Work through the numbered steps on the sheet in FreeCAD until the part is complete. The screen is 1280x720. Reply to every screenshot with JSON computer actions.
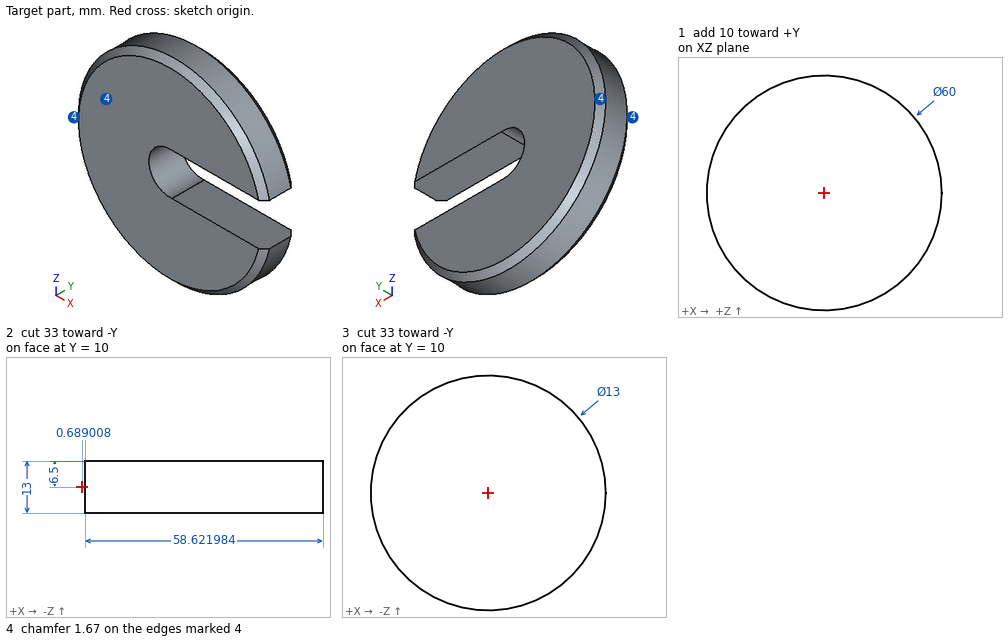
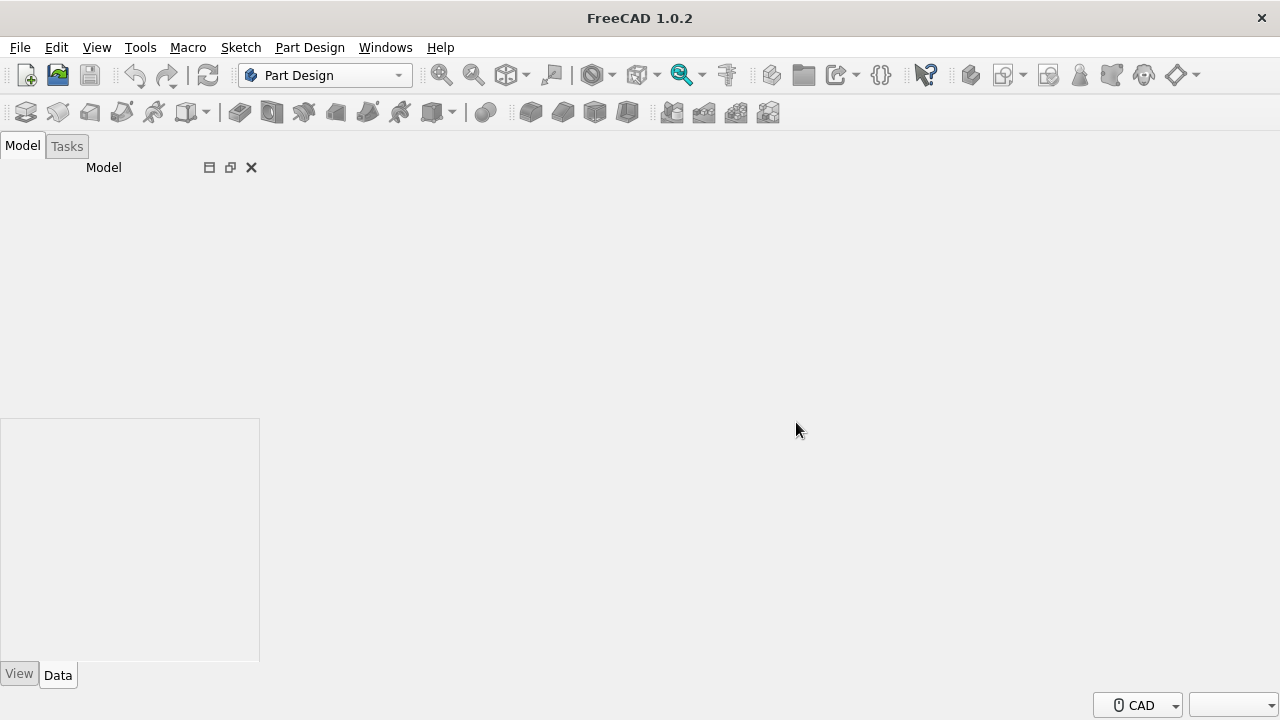
{"action": "left_click", "coordinate": [26, 76]}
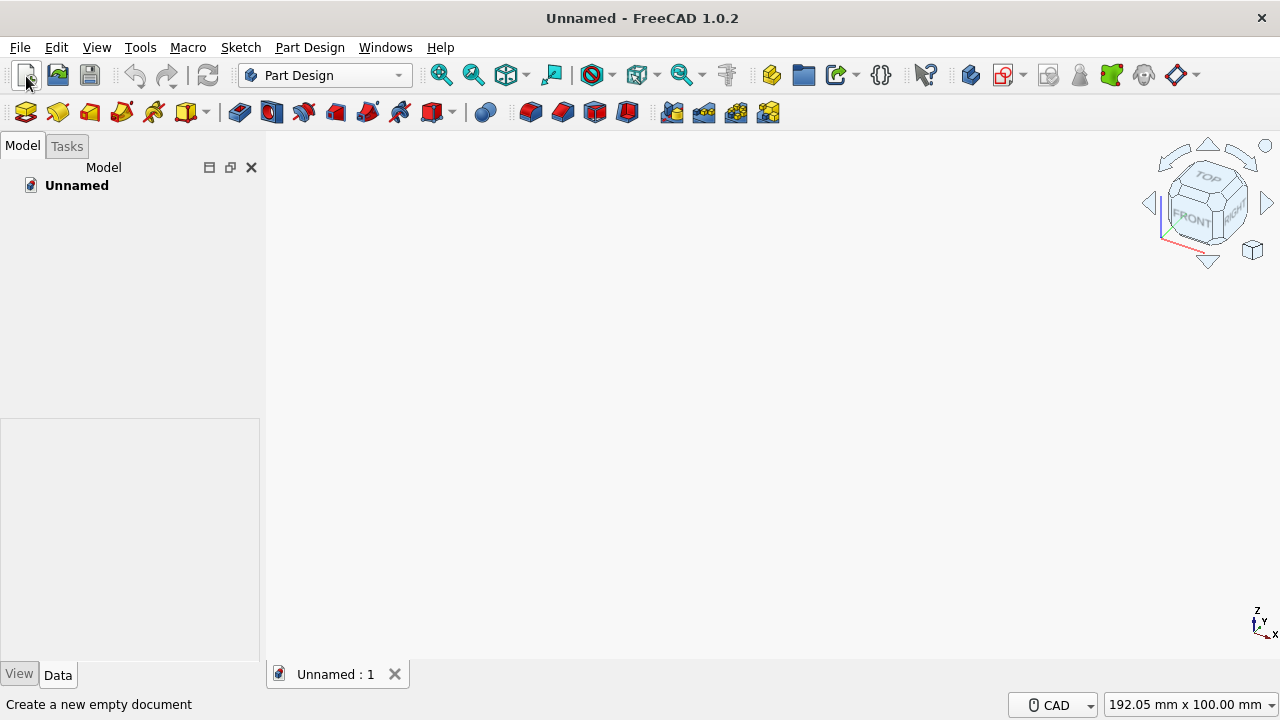
{"action": "left_click", "coordinate": [1004, 76]}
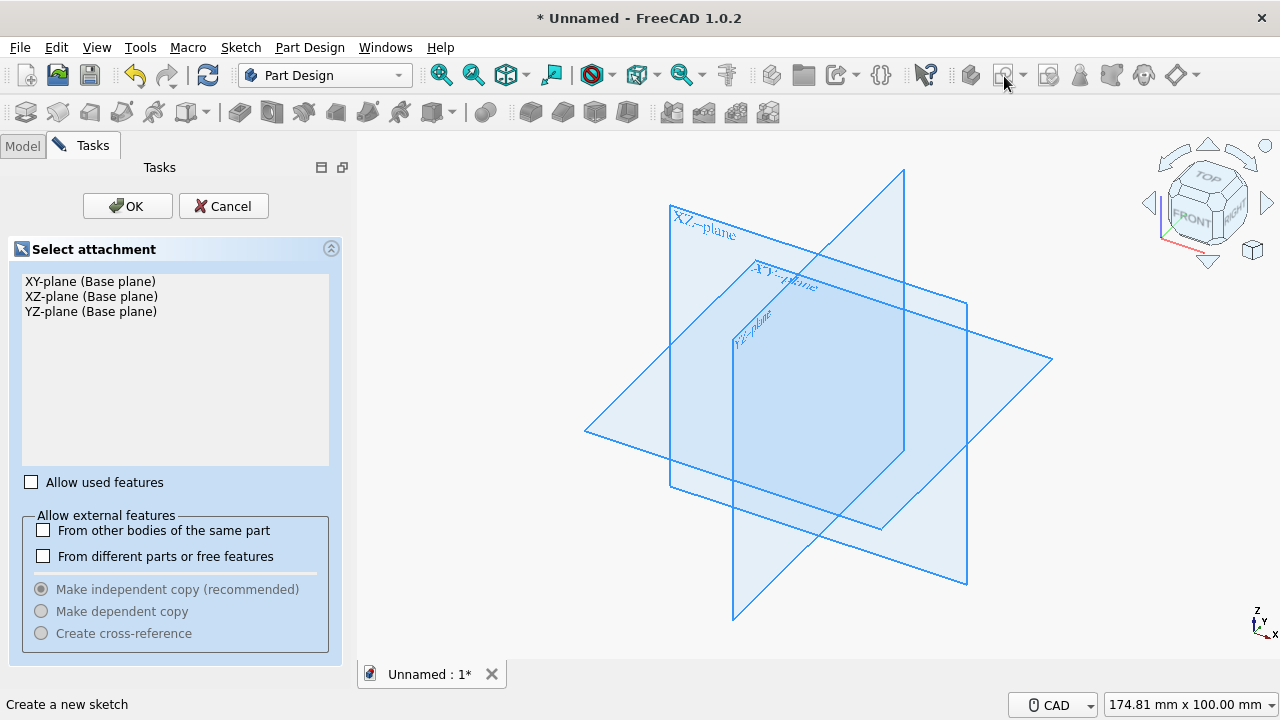
{"action": "left_click", "coordinate": [82, 296]}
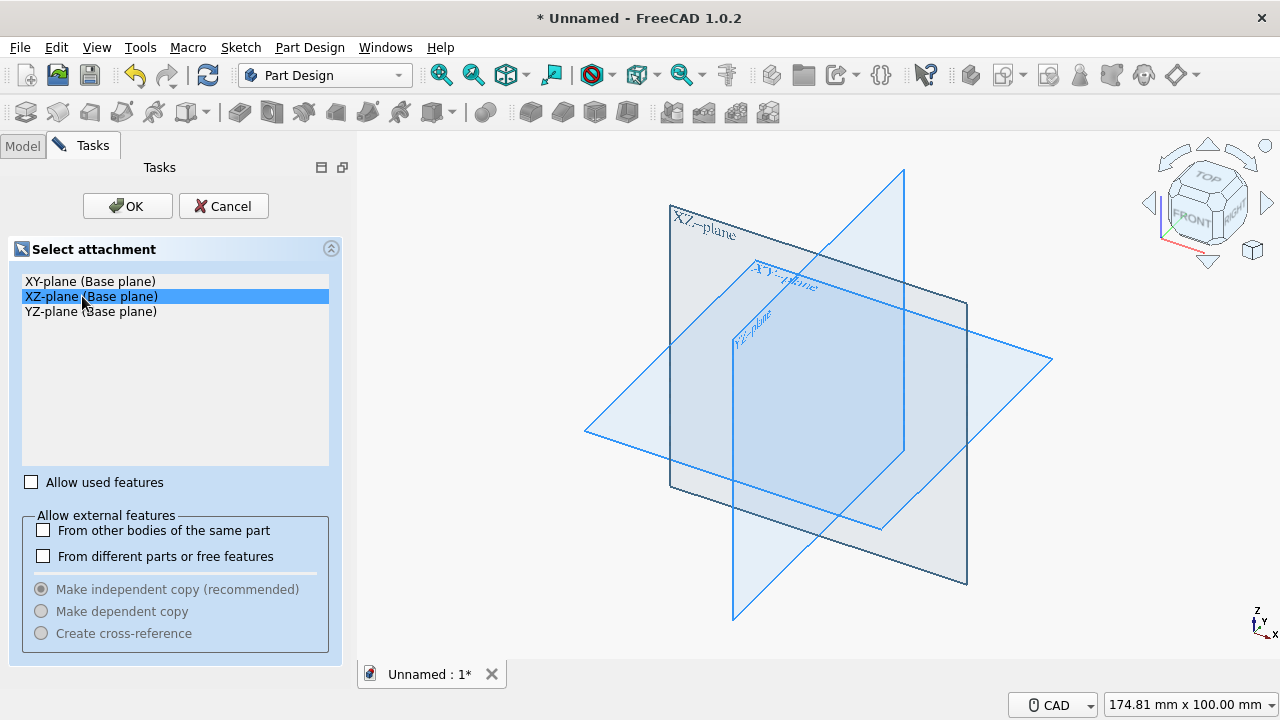
{"action": "left_click", "coordinate": [128, 206]}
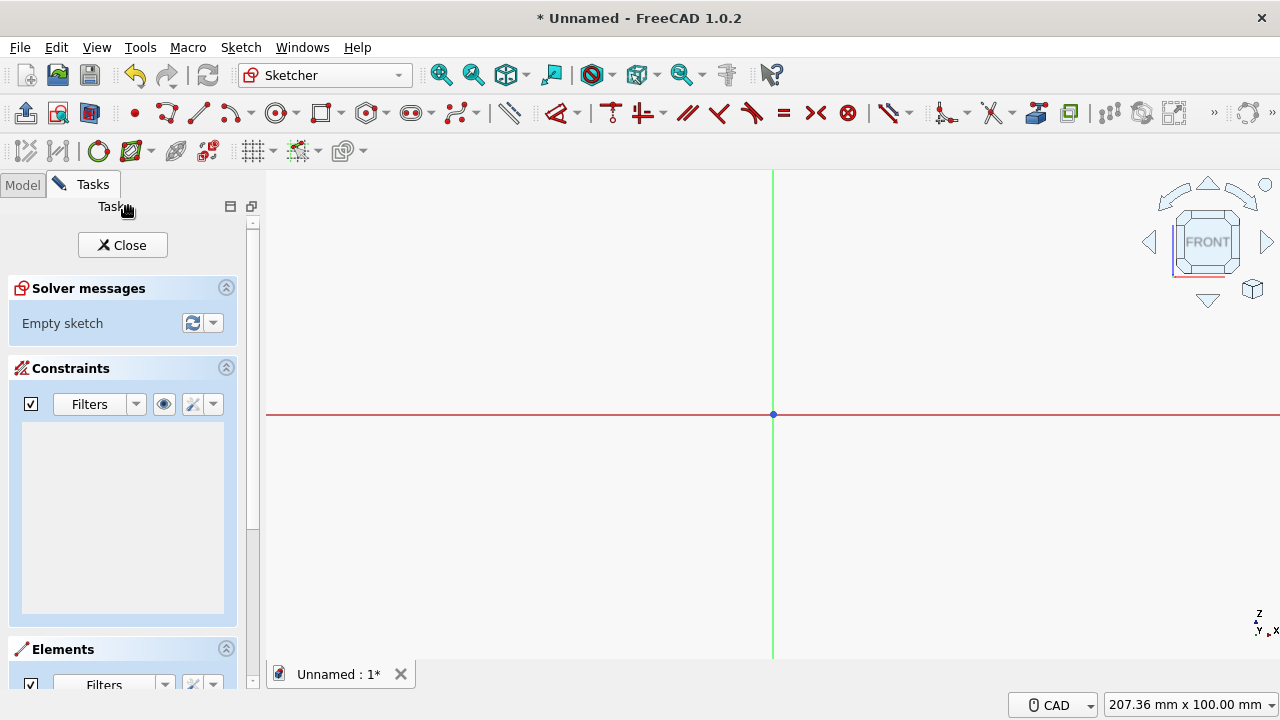
{"action": "key", "text": "g c"}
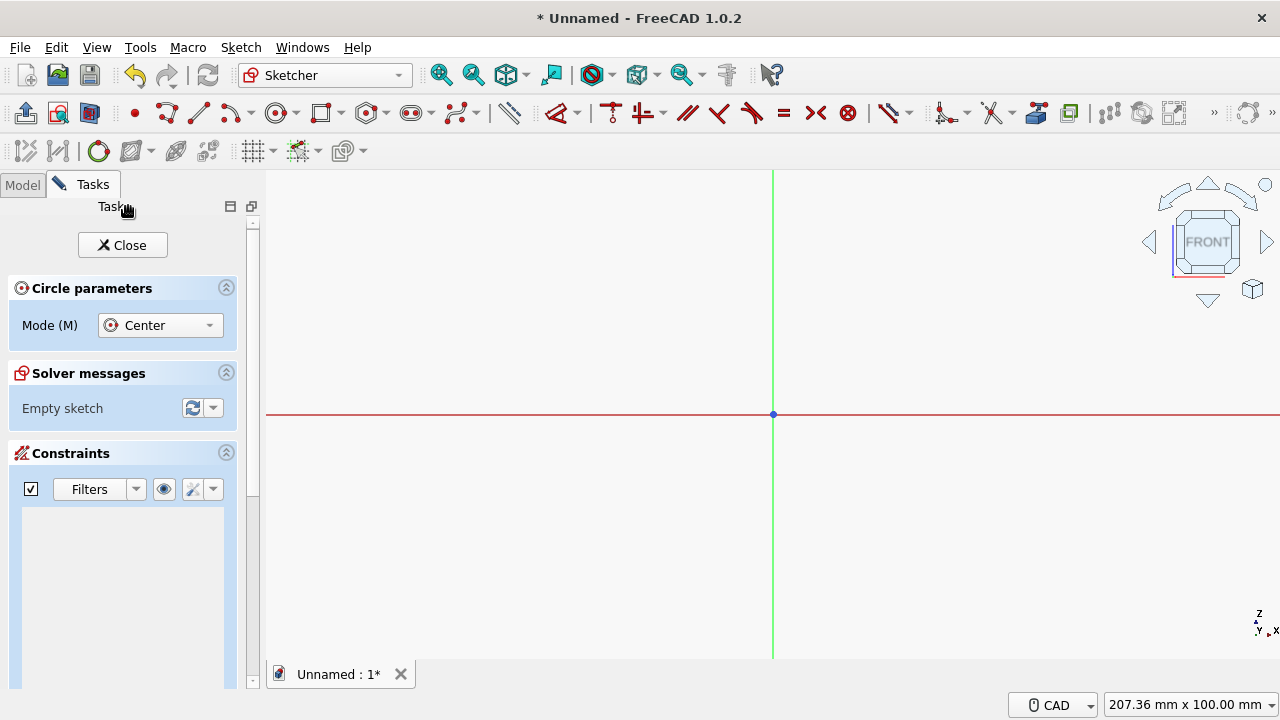
{"action": "left_click", "coordinate": [773, 414]}
{"action": "mouse_move", "coordinate": [877, 311]}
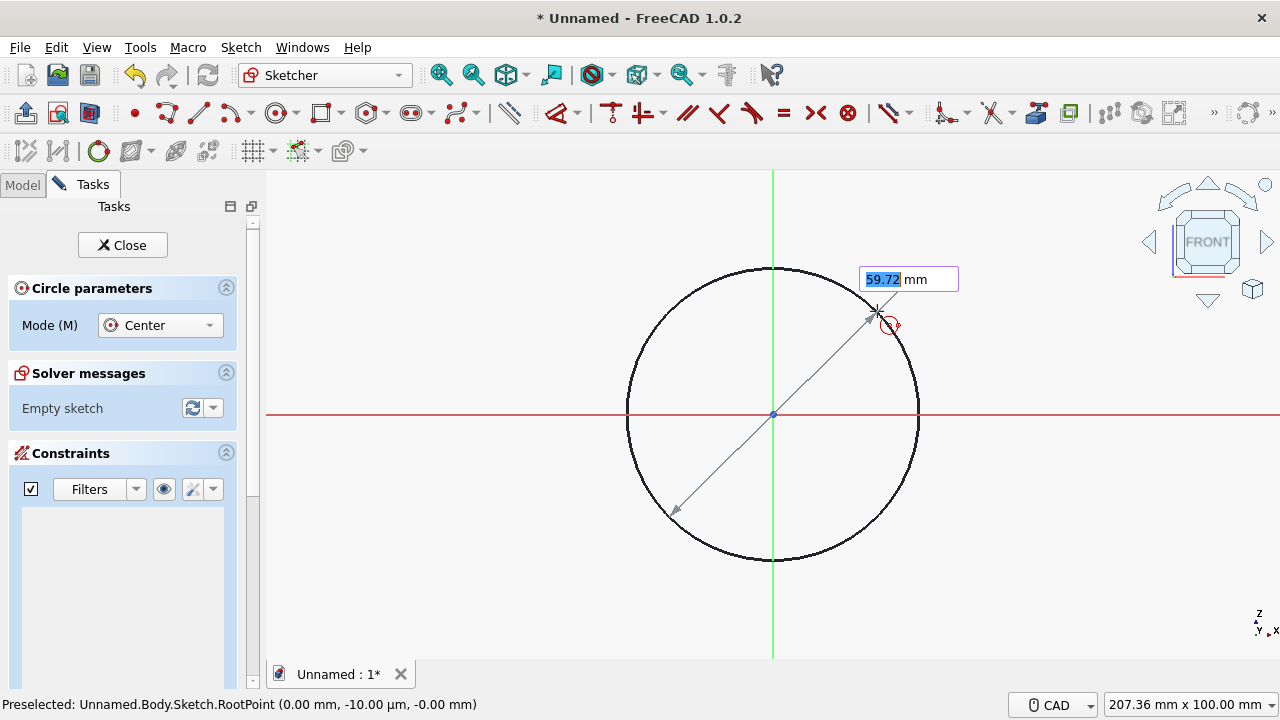
{"action": "type", "text": "60"}
{"action": "key", "text": "Return"}
{"action": "key", "text": "Escape"}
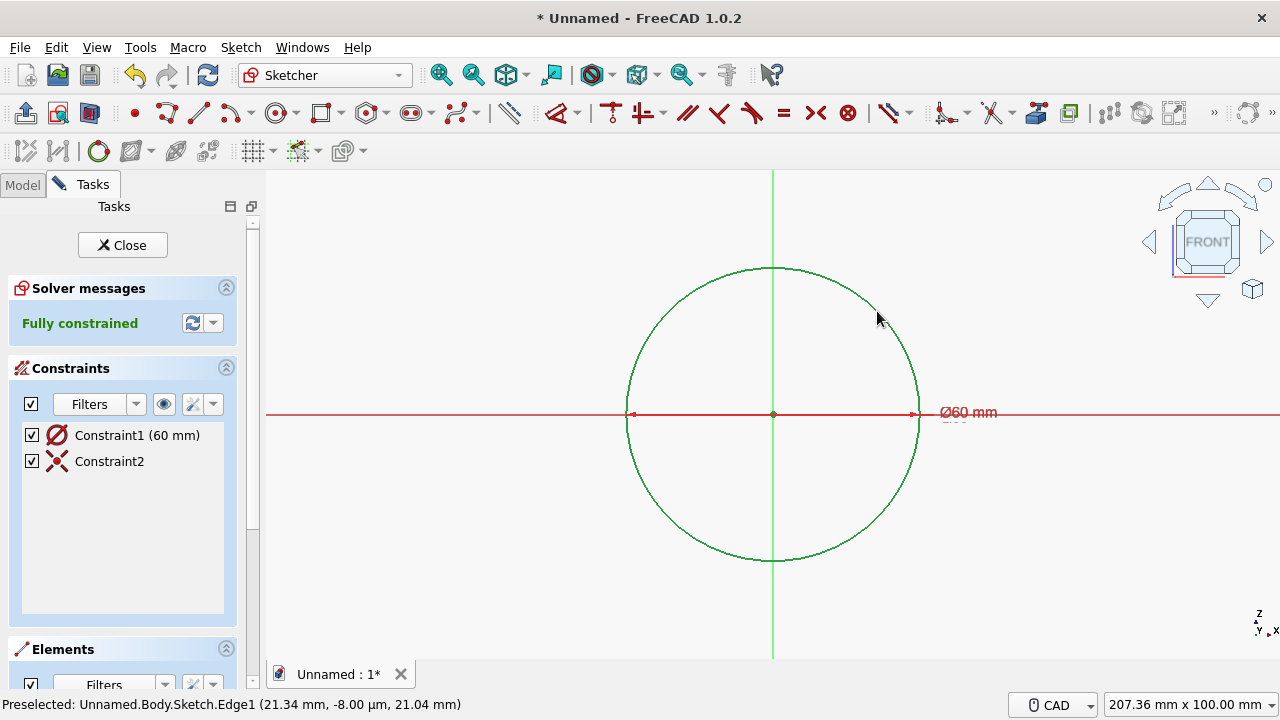
{"action": "left_click", "coordinate": [123, 245]}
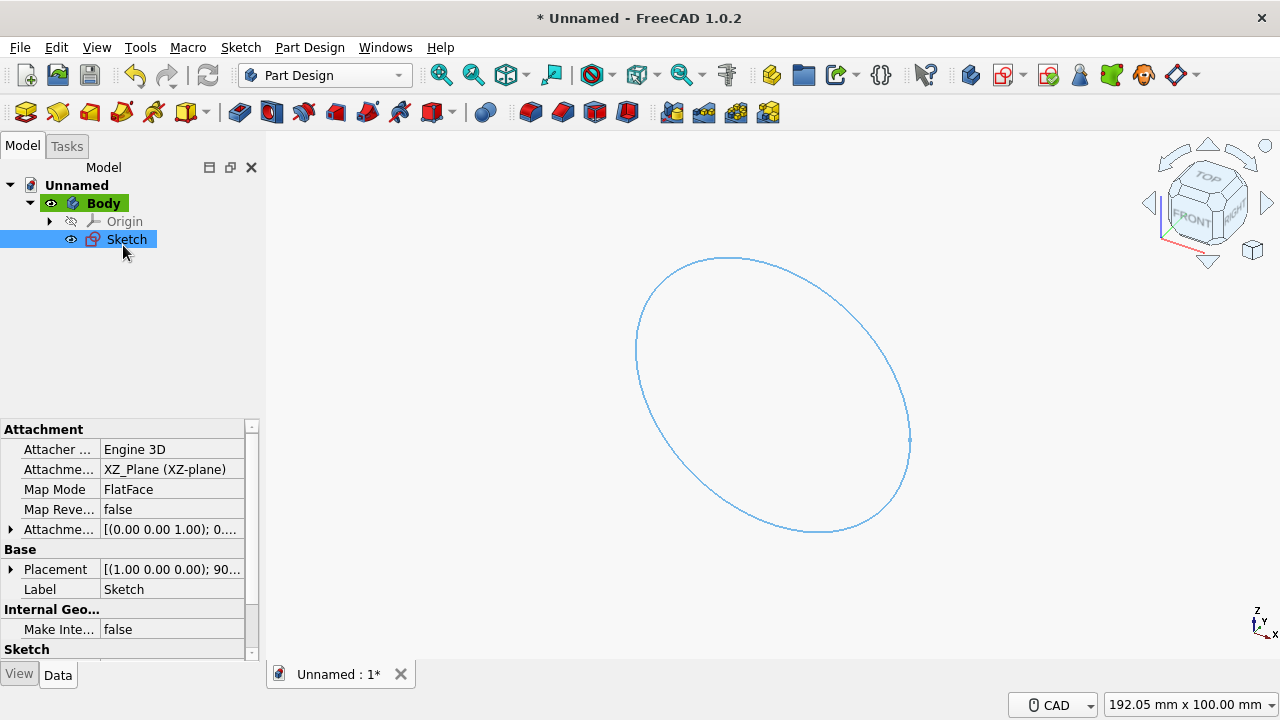
{"action": "left_click", "coordinate": [26, 112]}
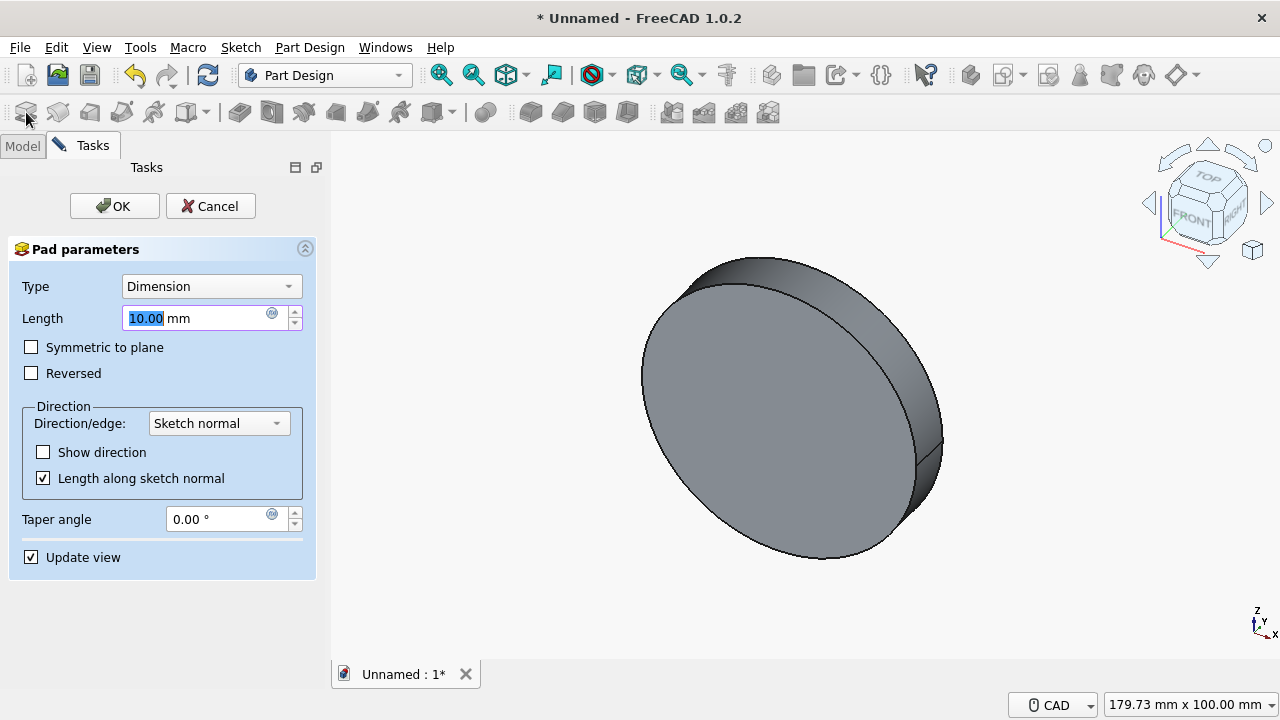
{"action": "type", "text": "10"}
{"action": "key", "text": "Tab"}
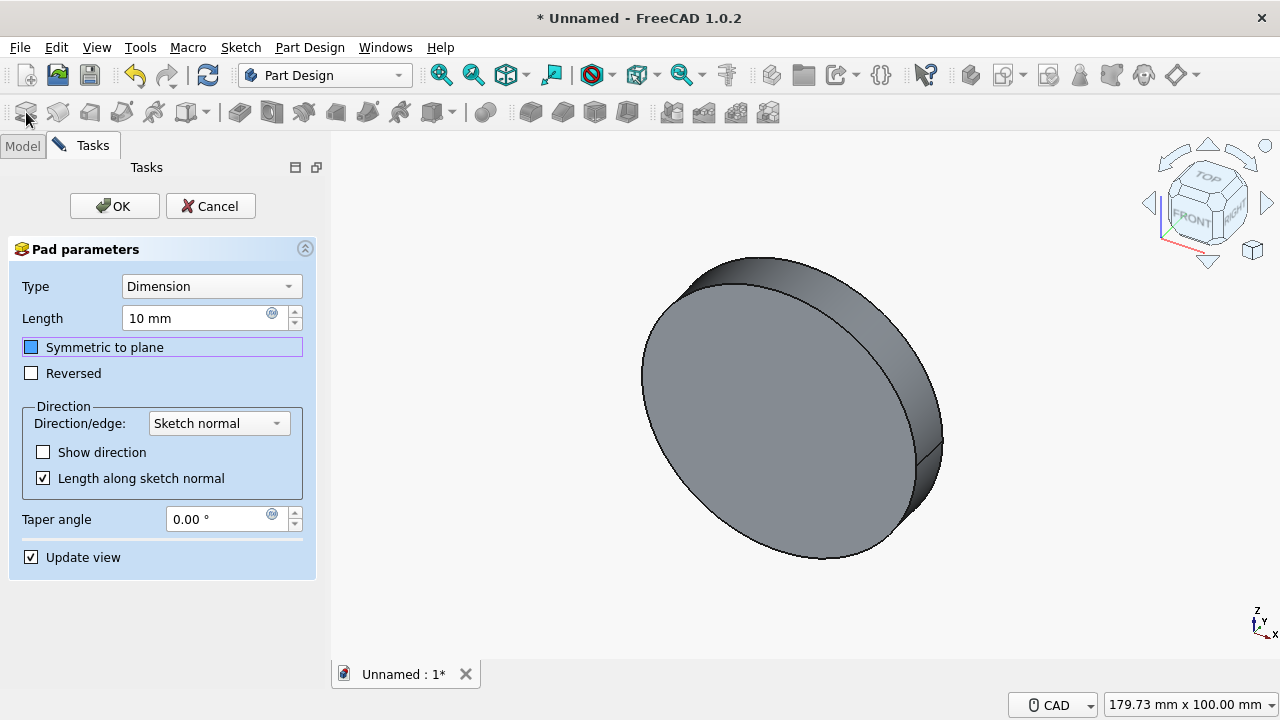
{"action": "left_click", "coordinate": [30, 373]}